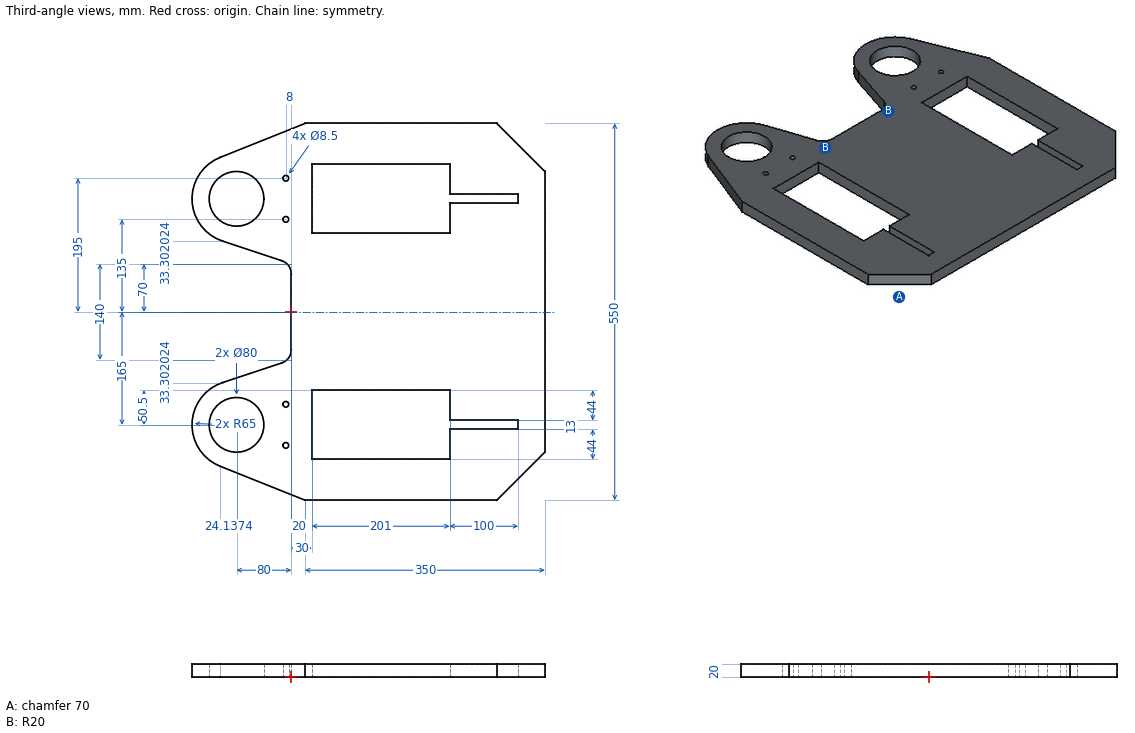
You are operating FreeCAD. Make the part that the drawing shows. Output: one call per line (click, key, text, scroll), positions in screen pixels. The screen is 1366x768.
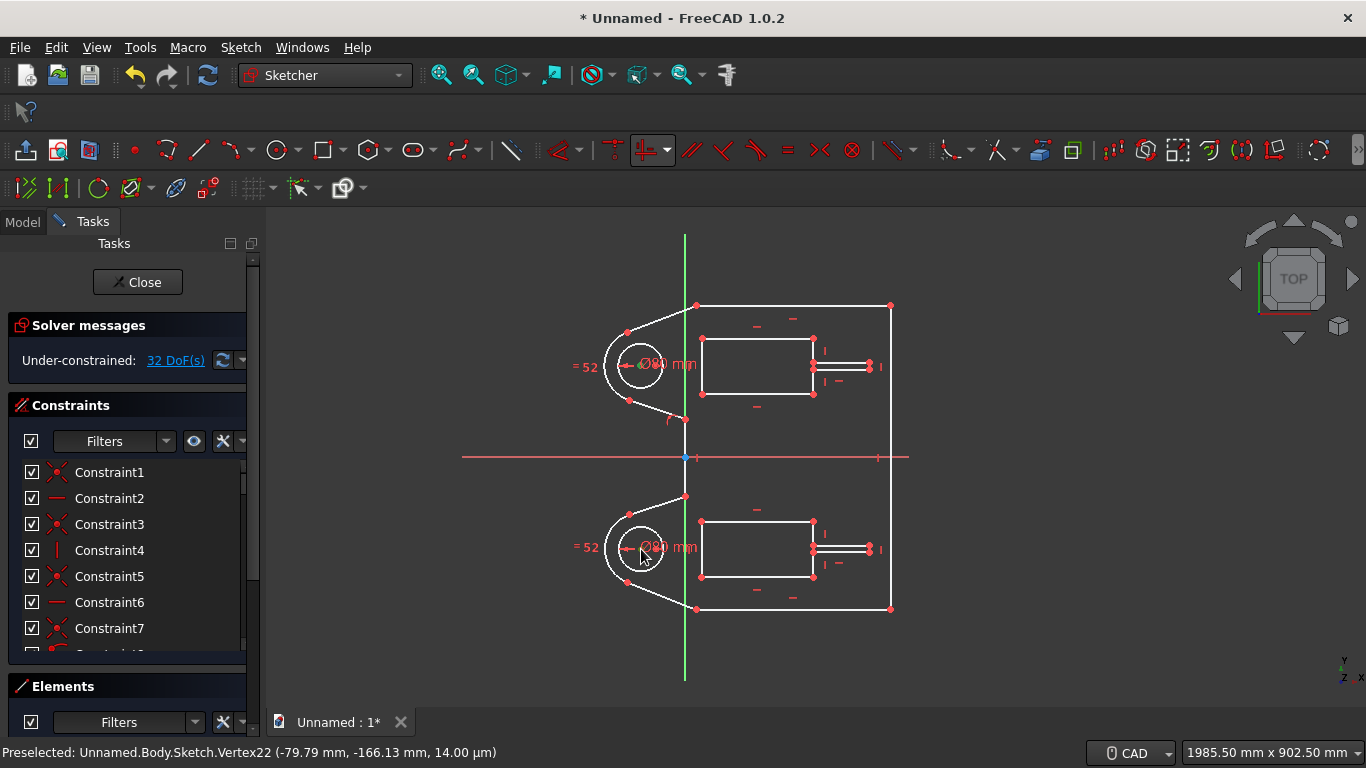
click(488, 457)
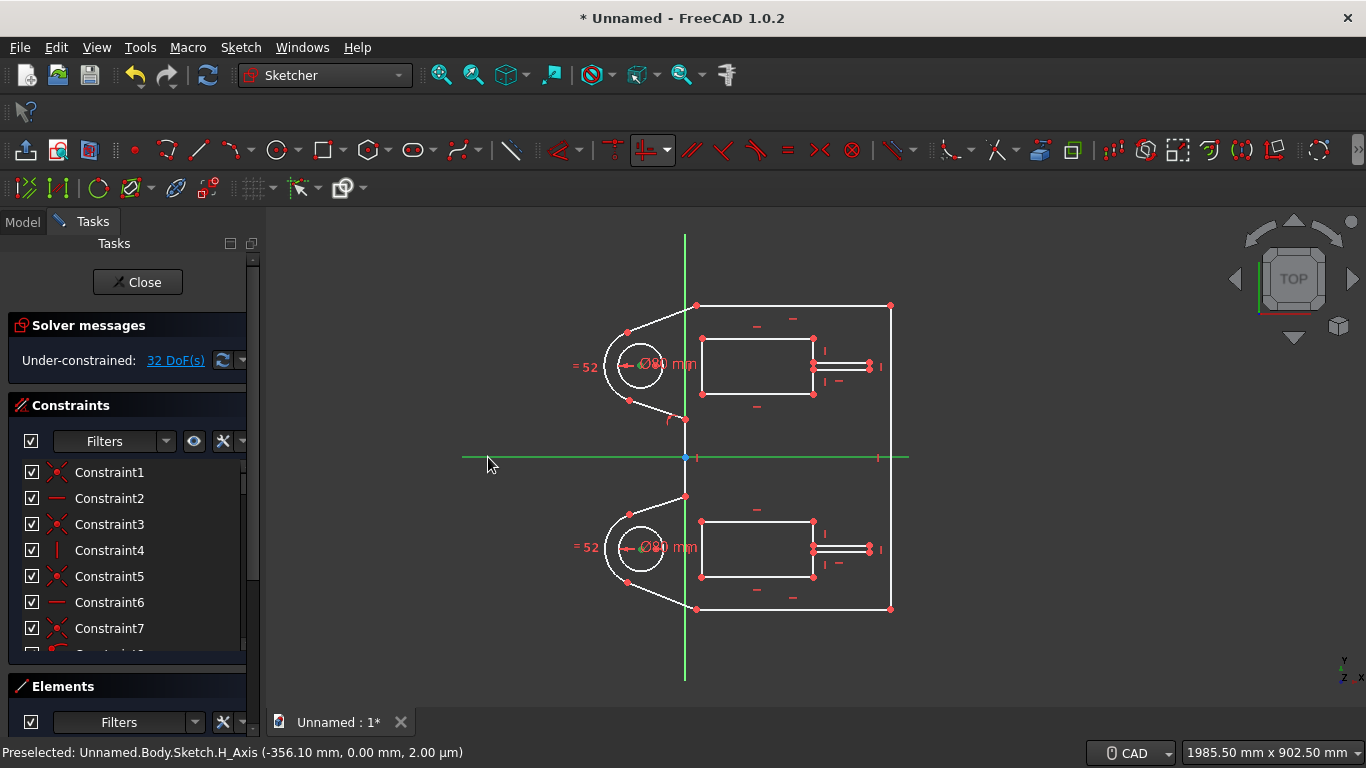
key(s)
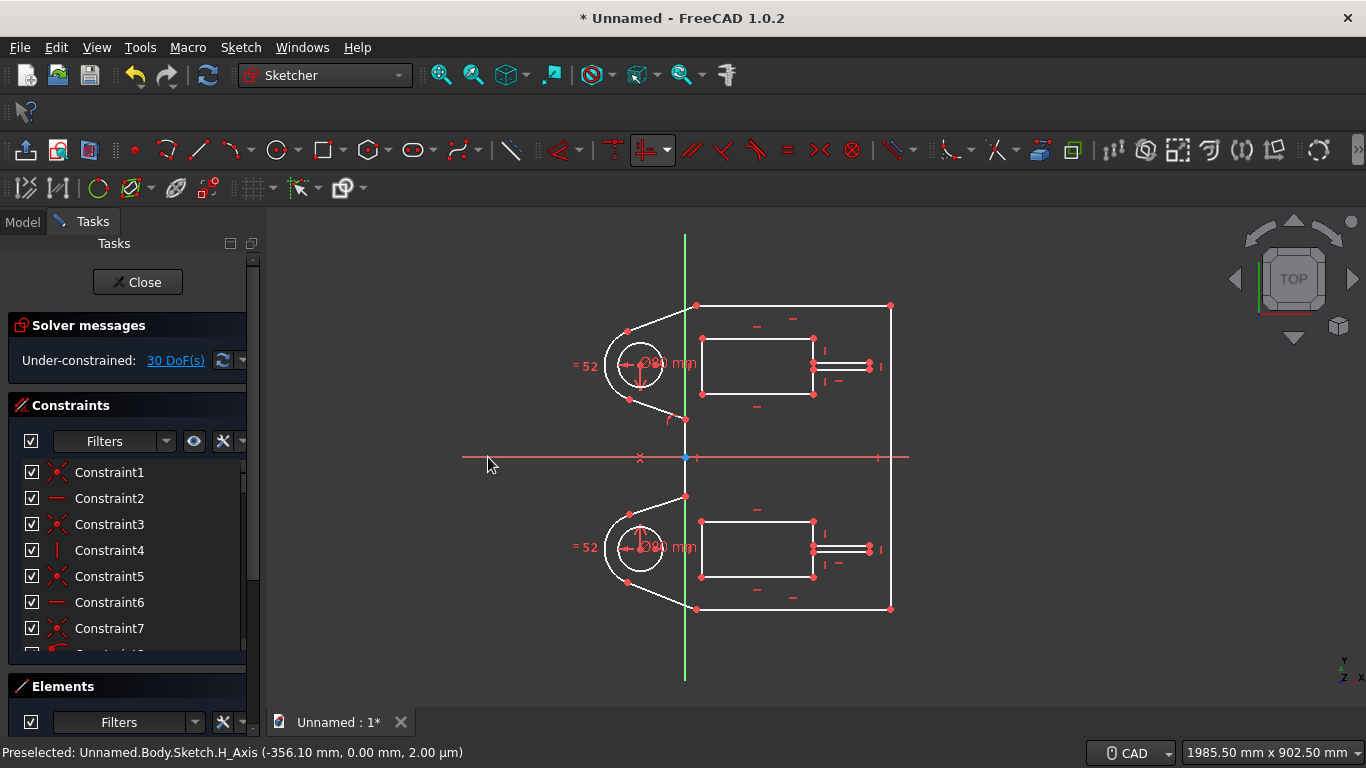
click(696, 610)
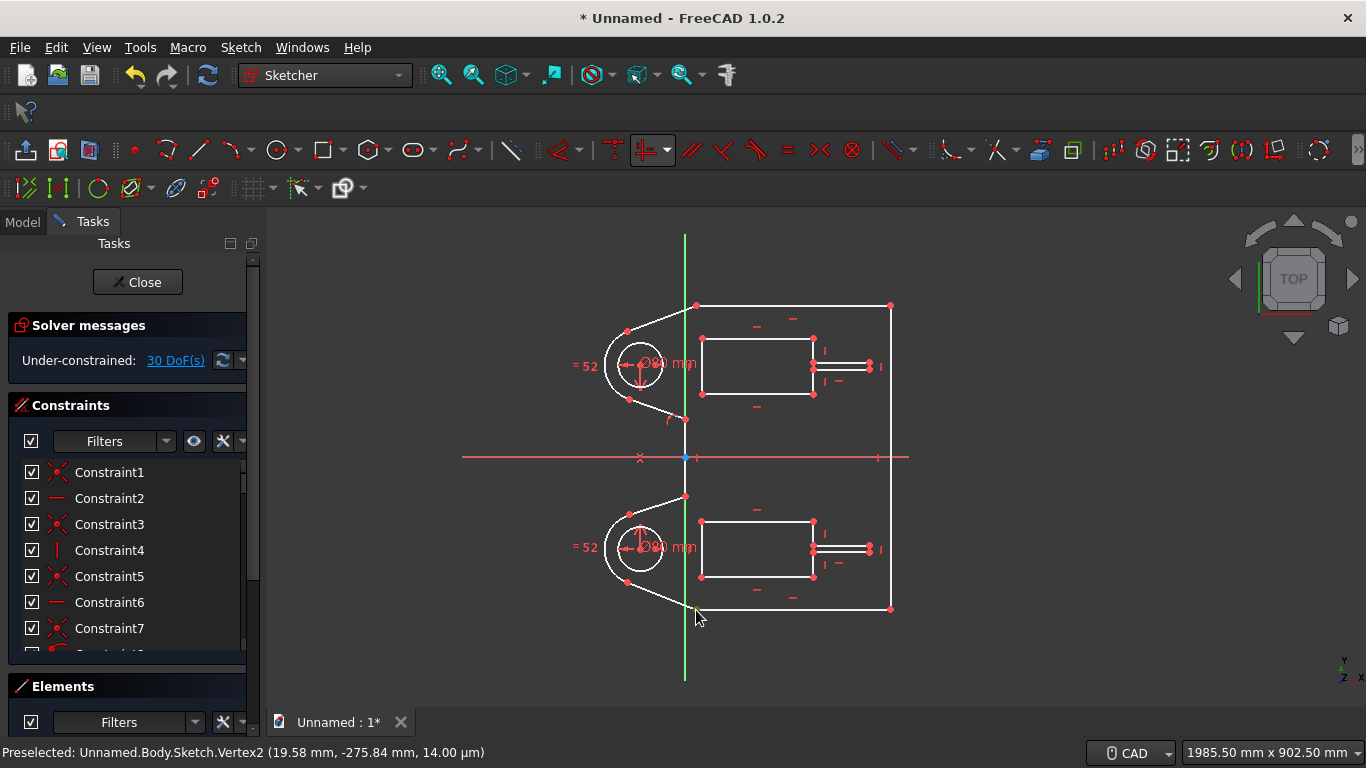
click(696, 306)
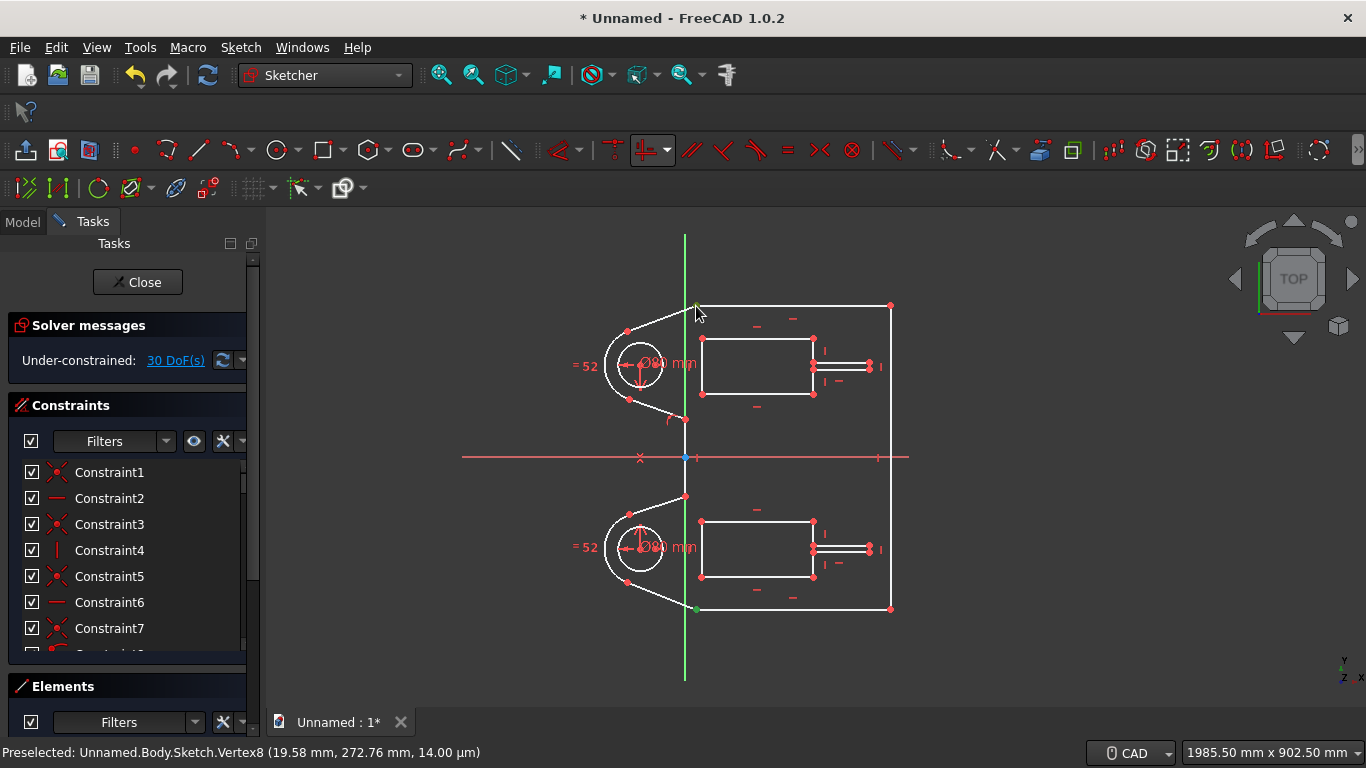
click(488, 457)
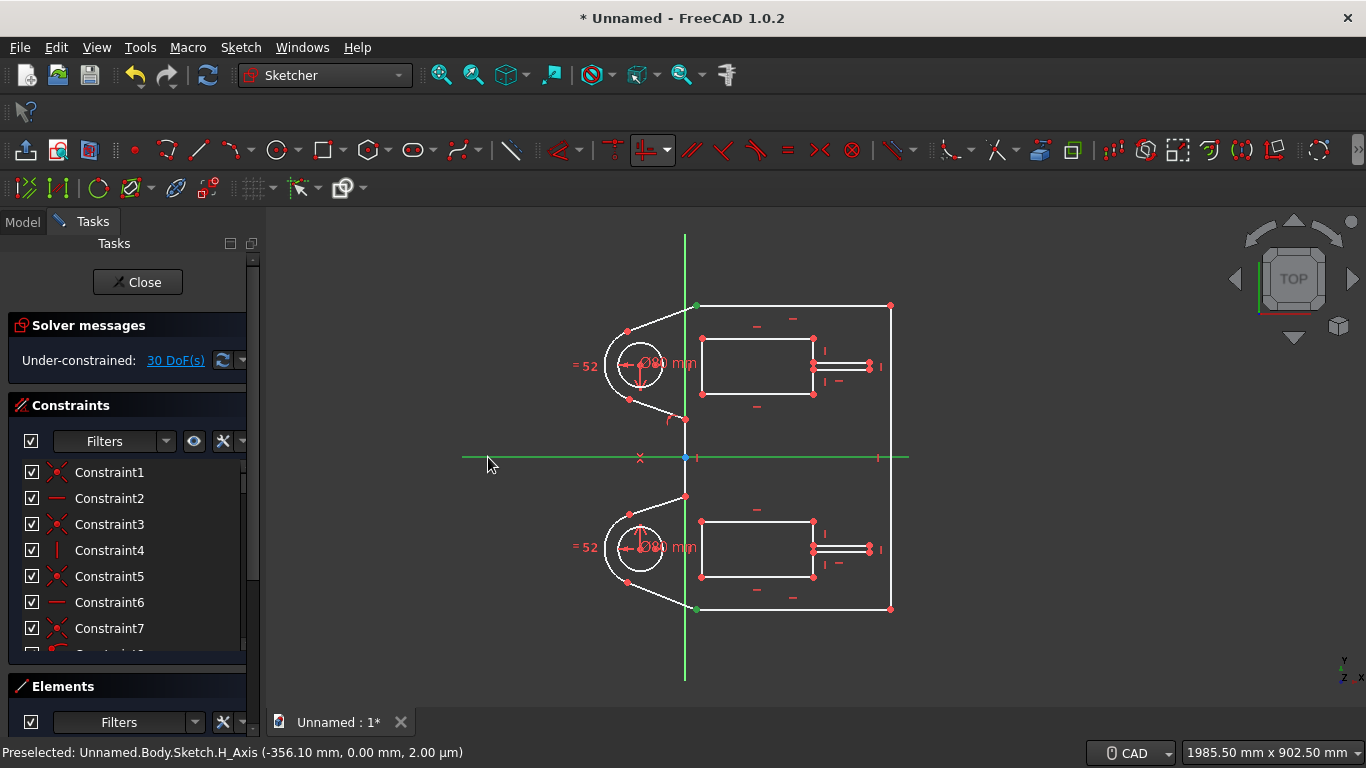
key(s)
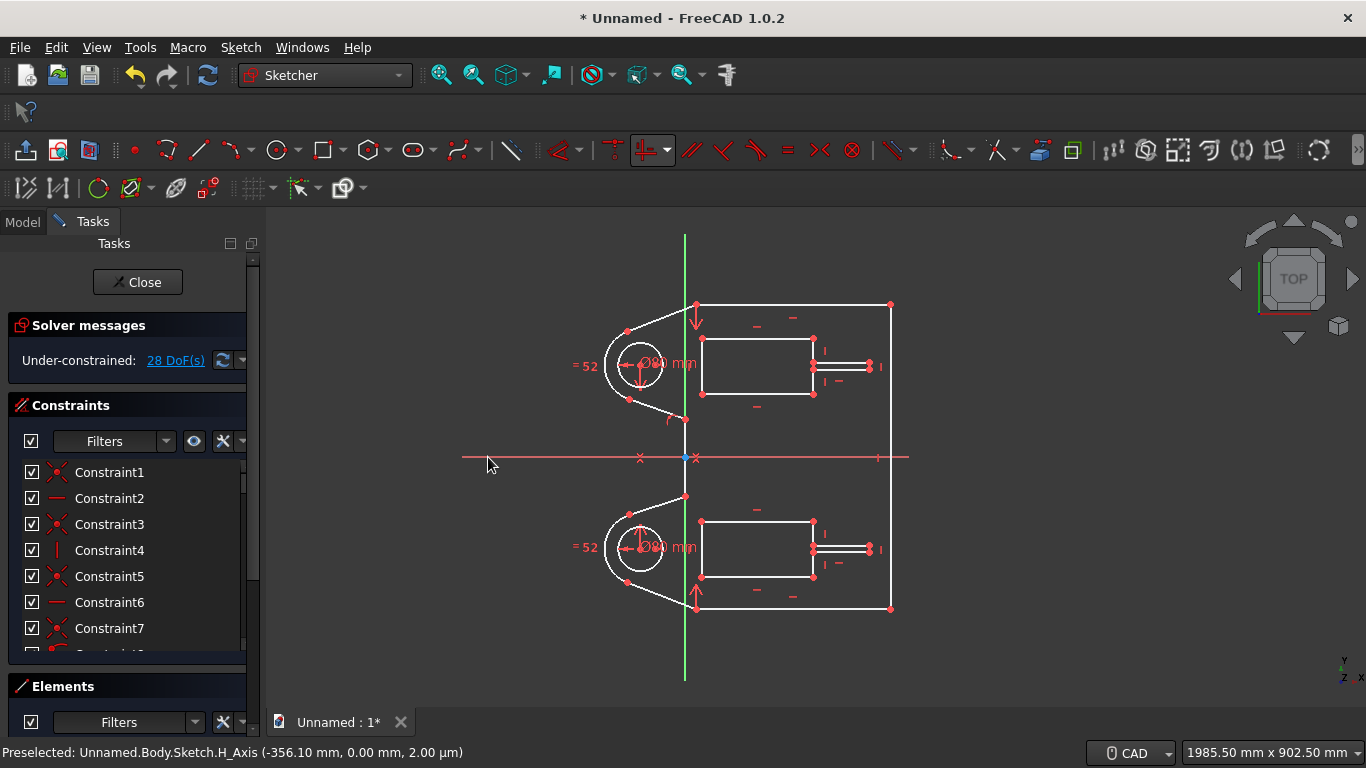
click(702, 522)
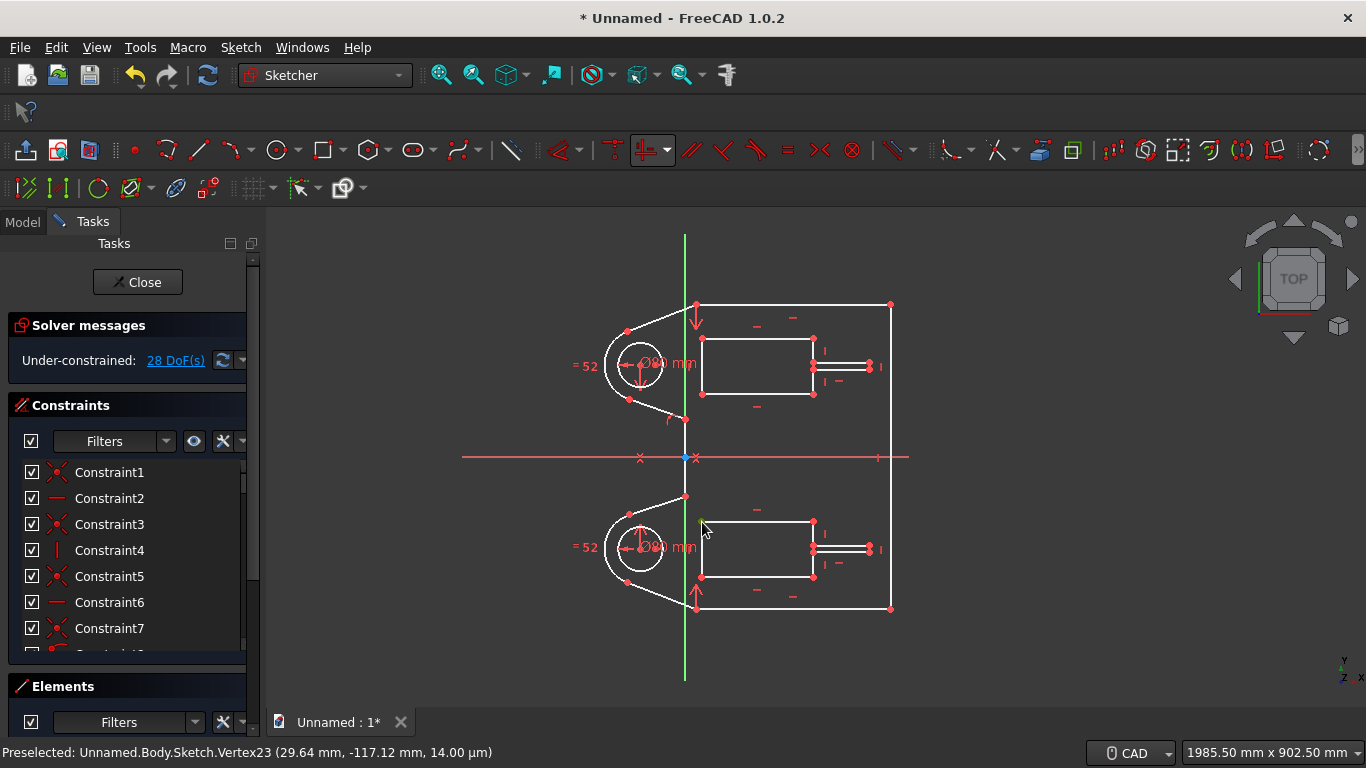
click(702, 394)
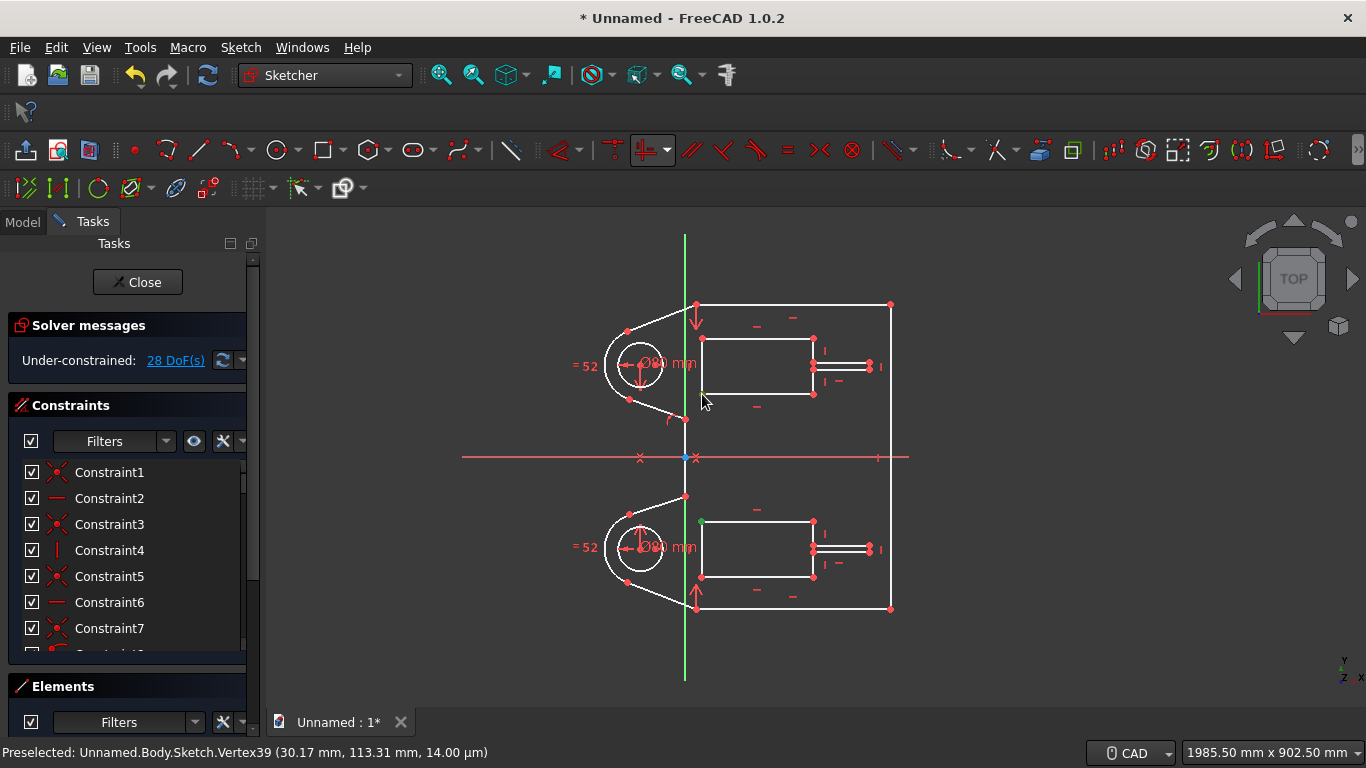
click(488, 457)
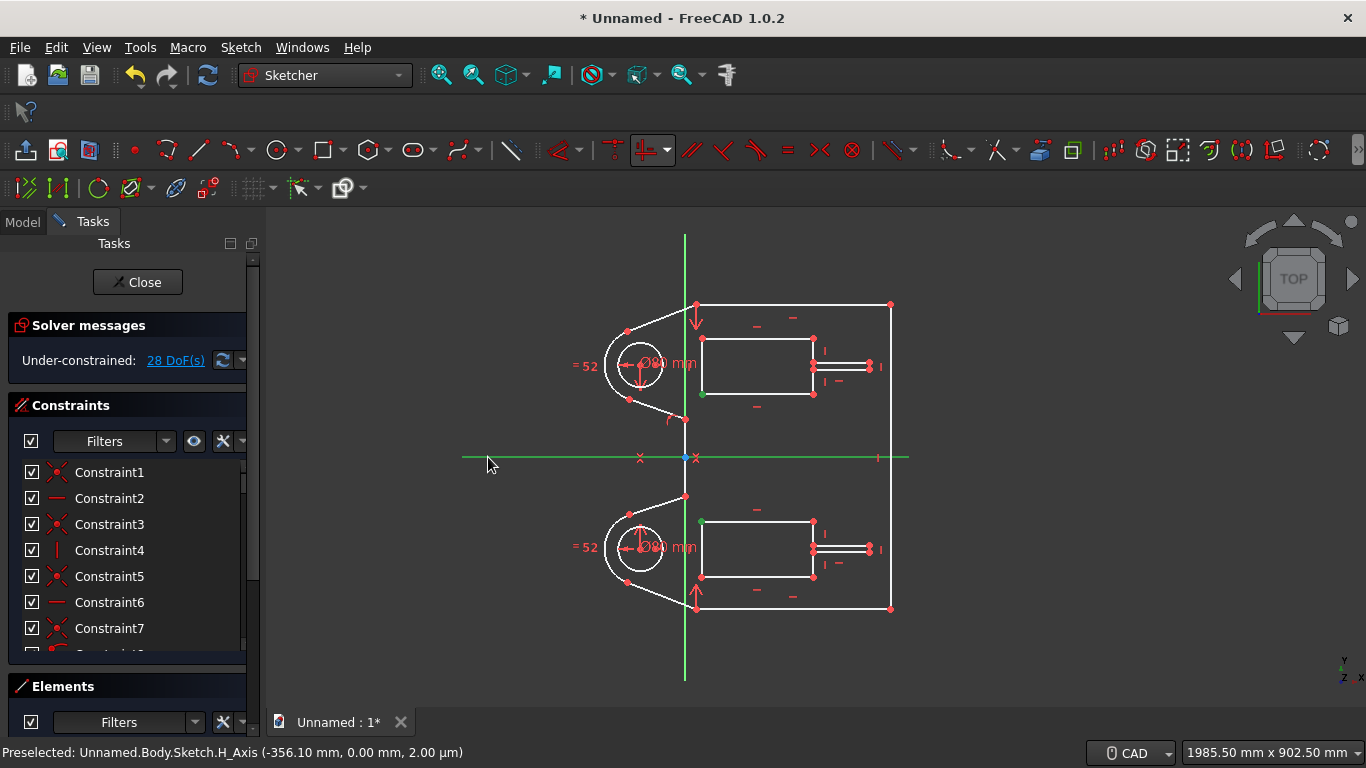
key(s)